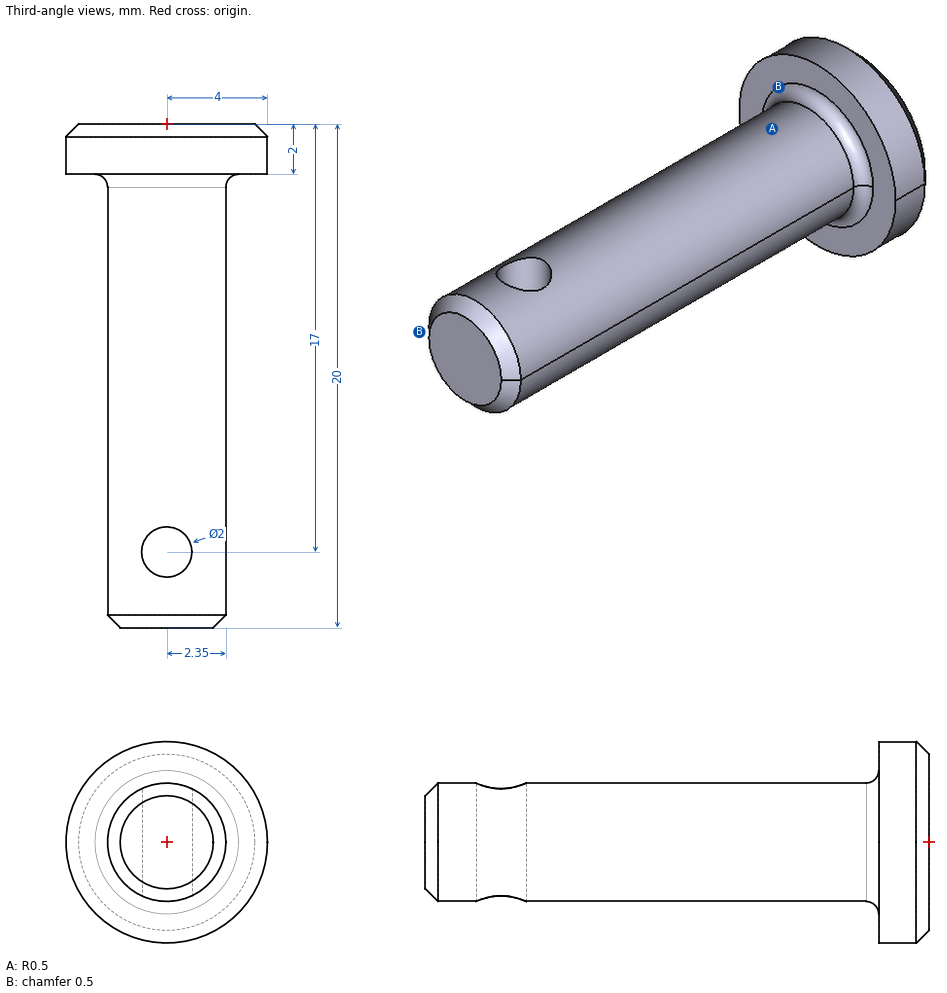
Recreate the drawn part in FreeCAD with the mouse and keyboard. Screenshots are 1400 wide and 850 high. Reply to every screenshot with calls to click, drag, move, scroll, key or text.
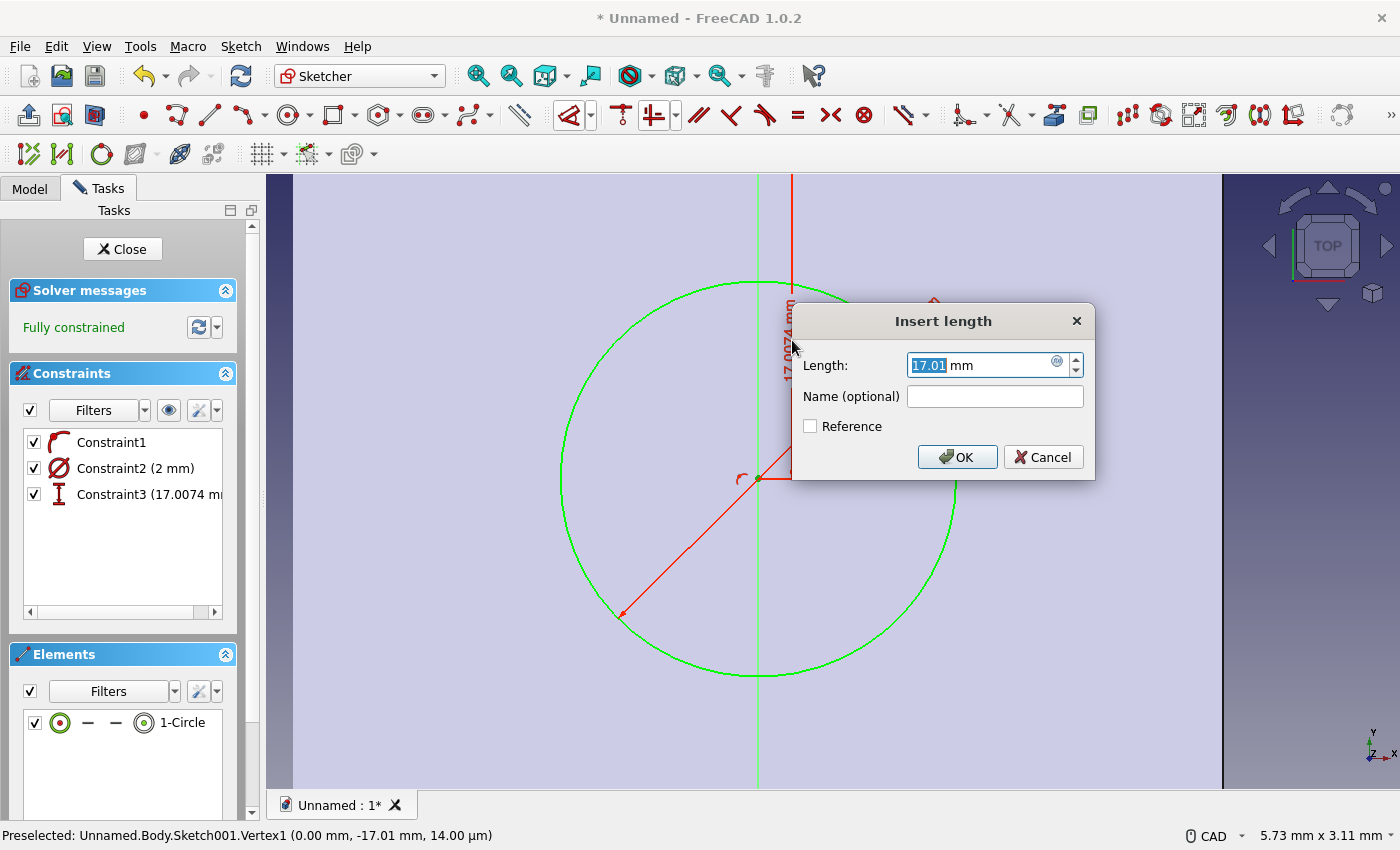
text(17)
key(Return)
key(Escape)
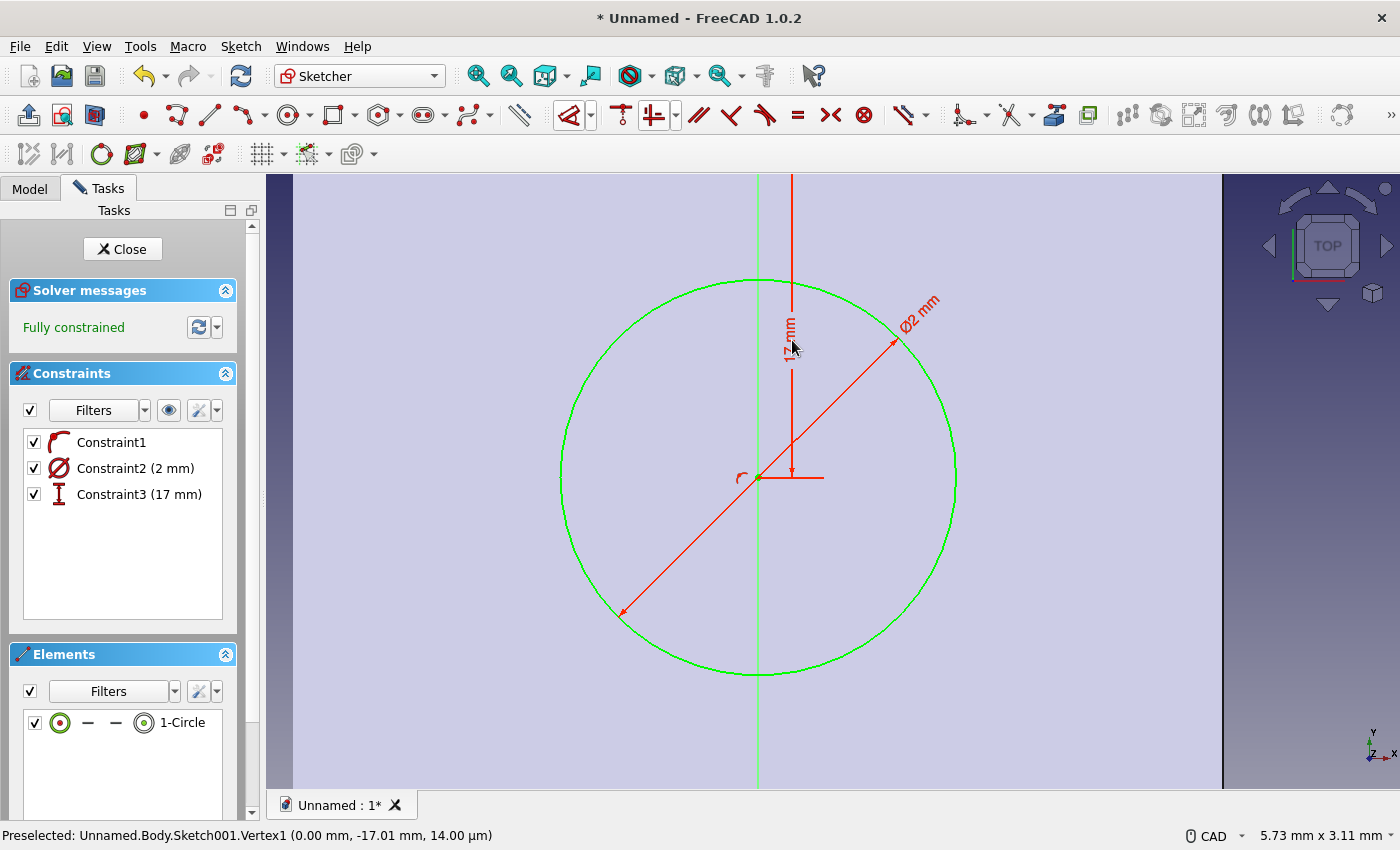
click(123, 249)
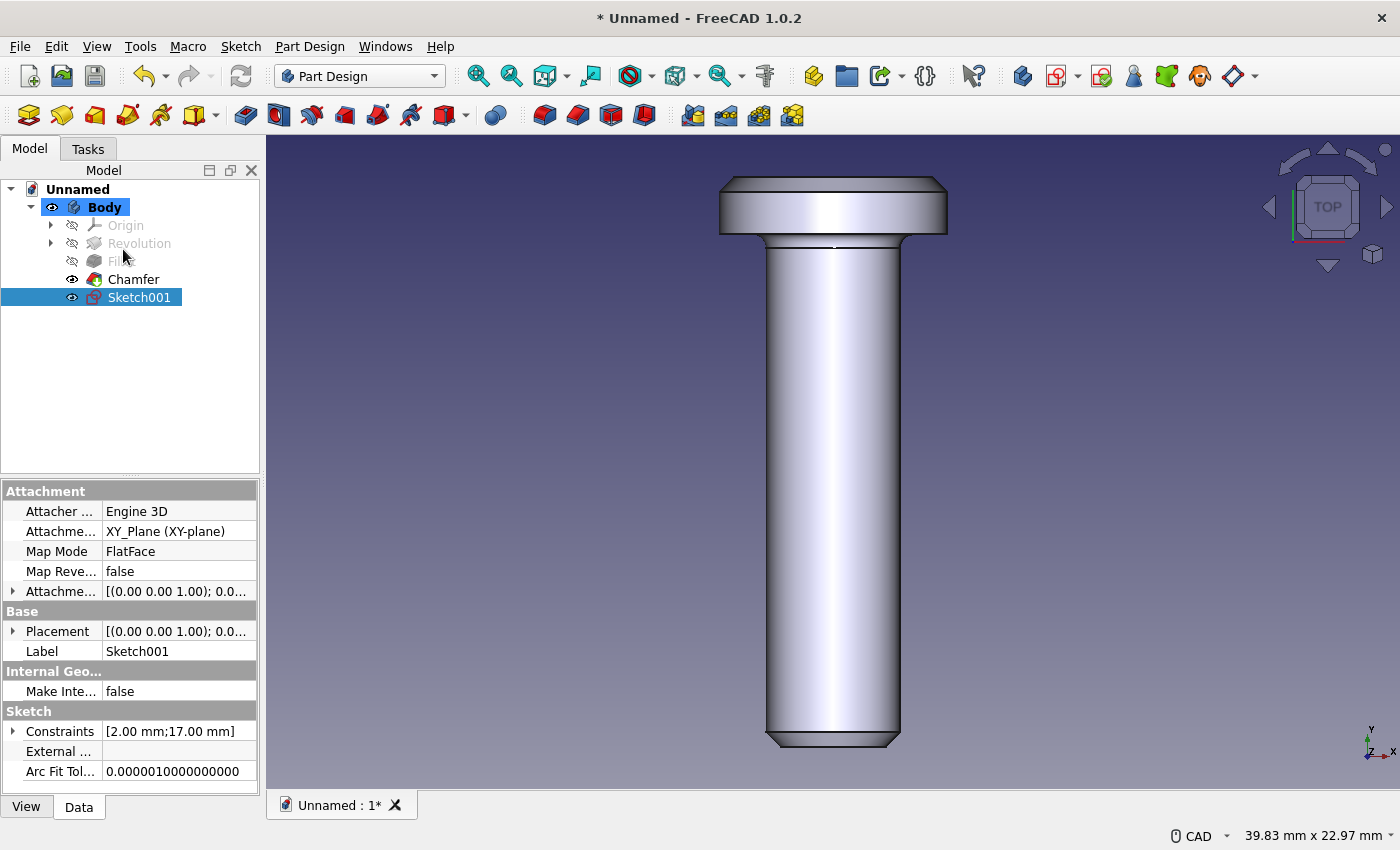
click(246, 116)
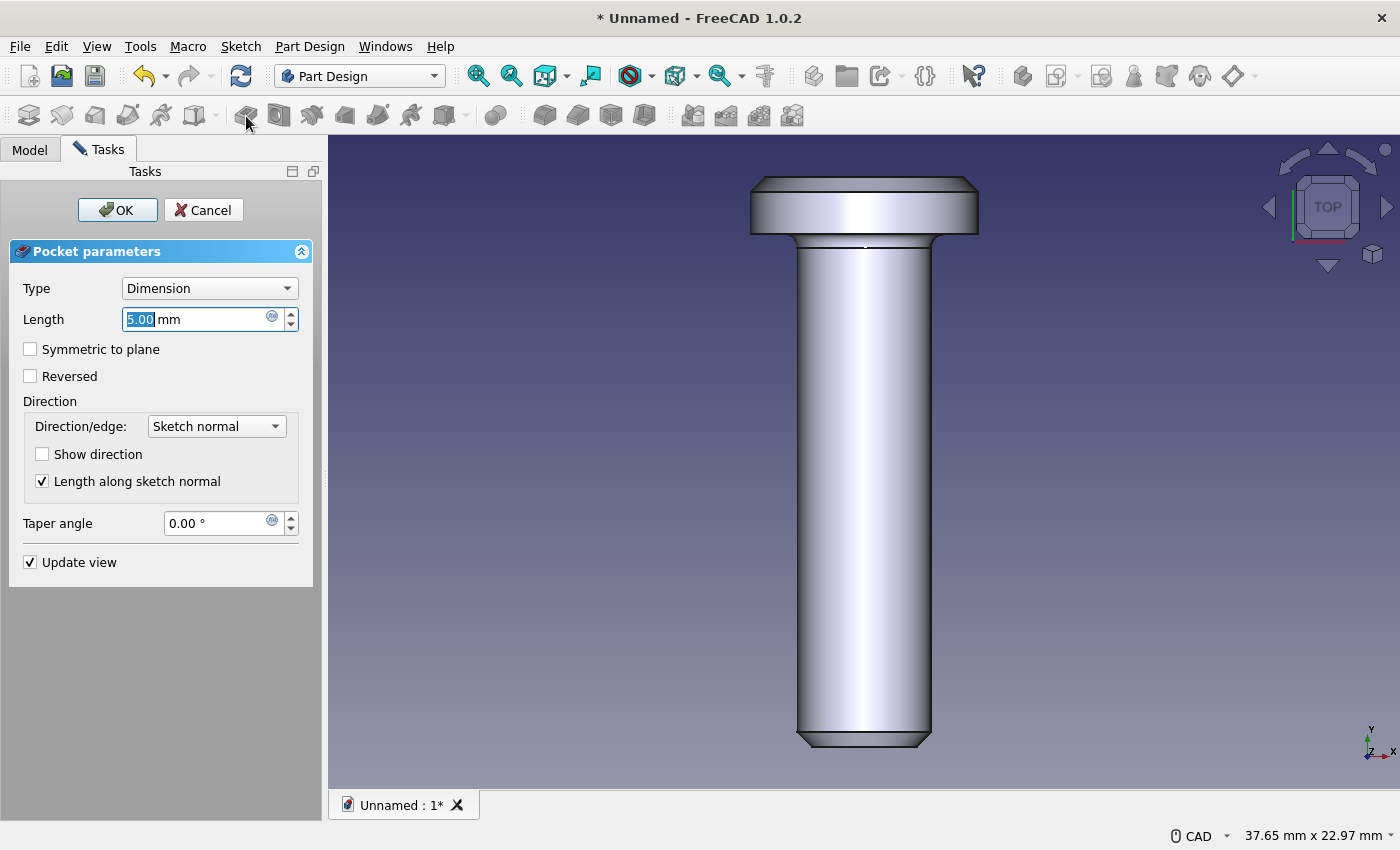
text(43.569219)
key(Tab)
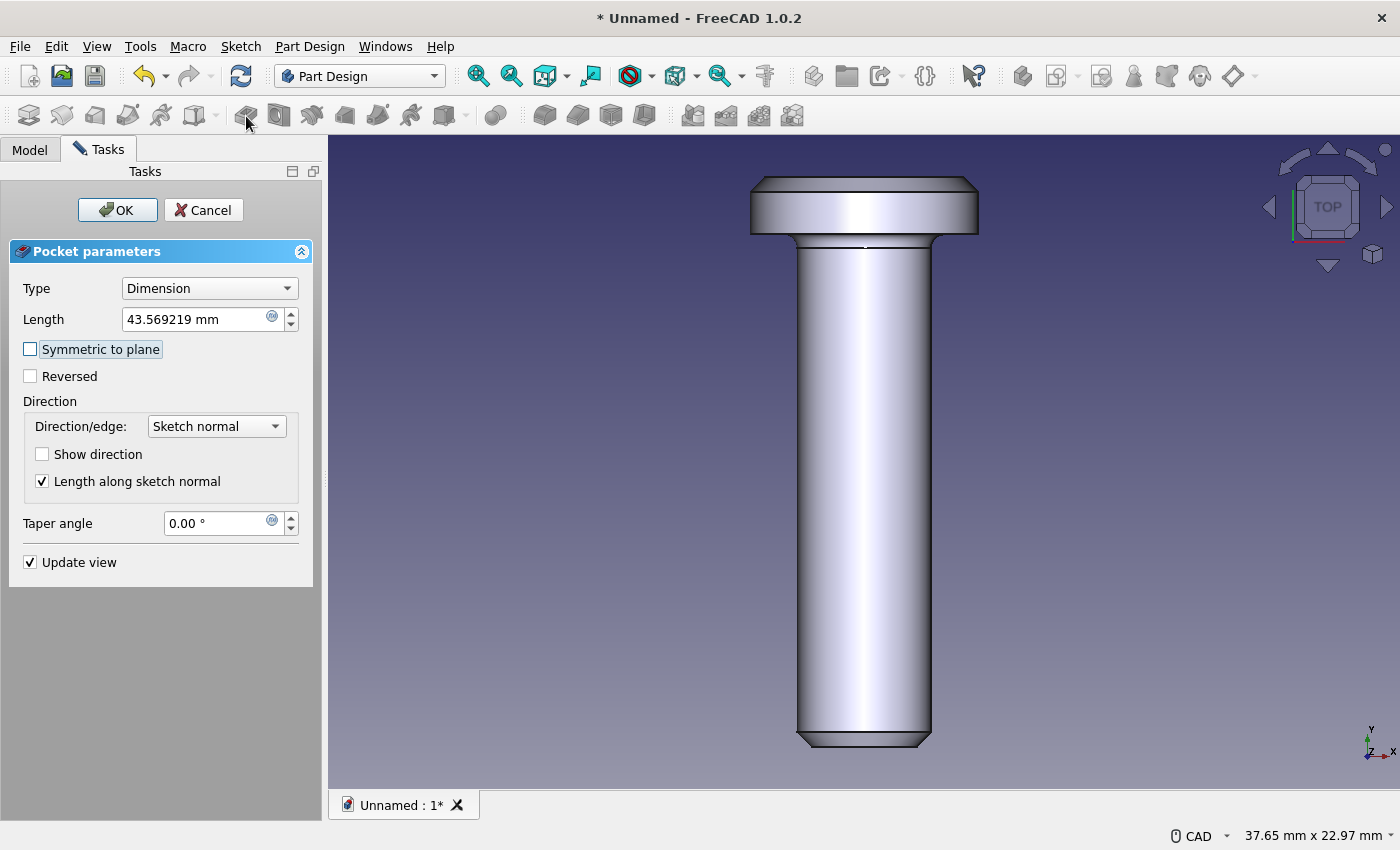
click(31, 349)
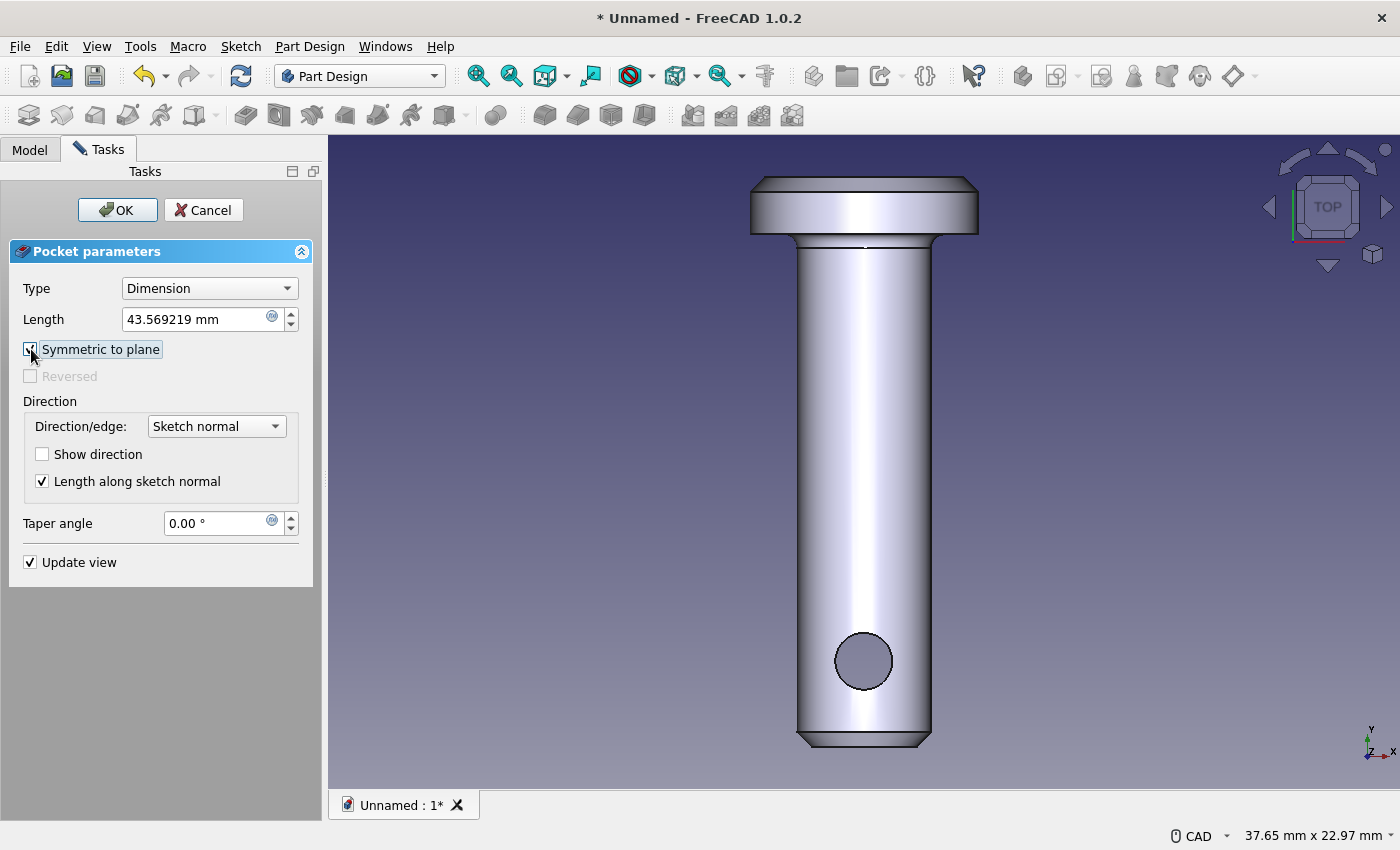
click(118, 210)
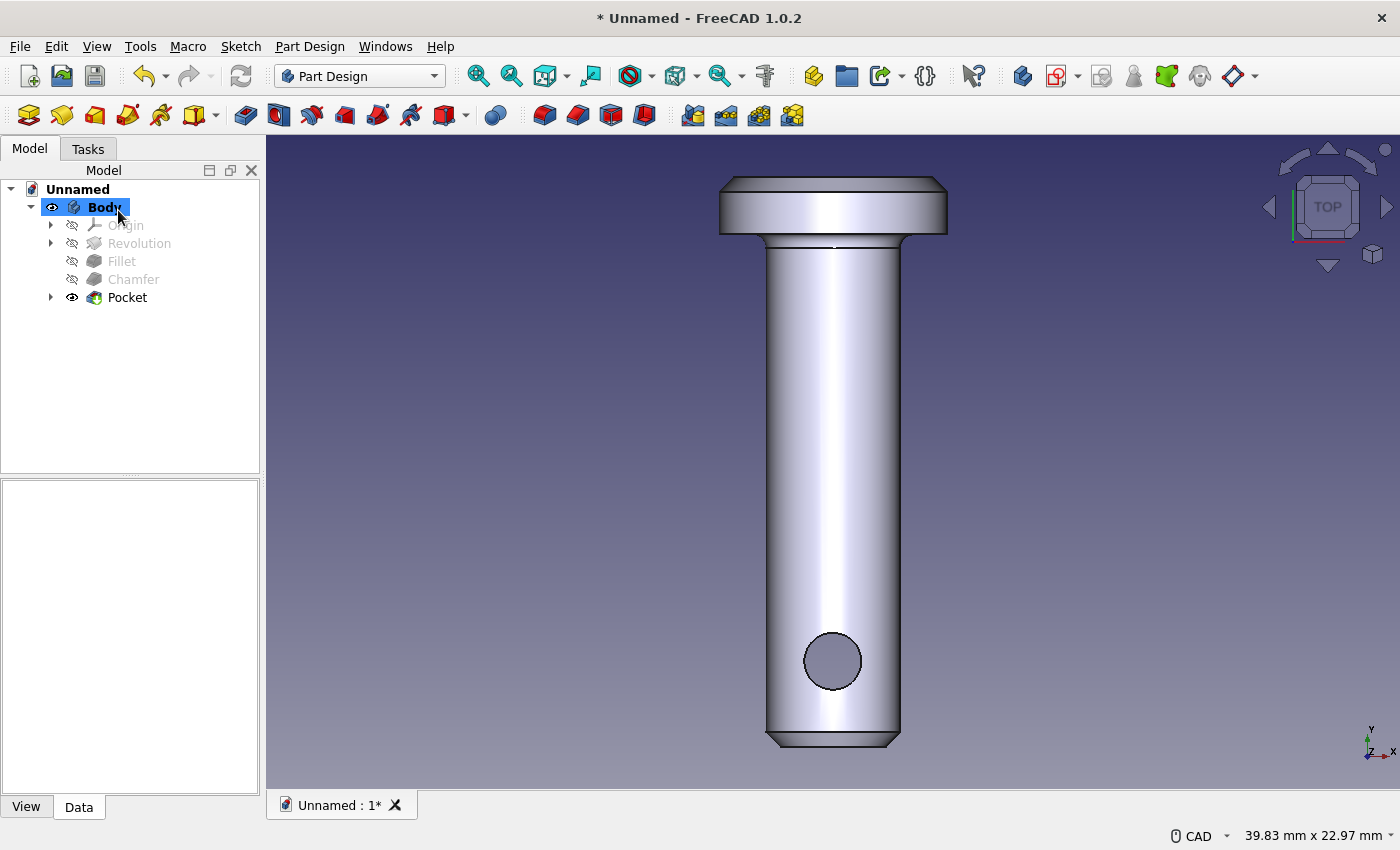
key(0)